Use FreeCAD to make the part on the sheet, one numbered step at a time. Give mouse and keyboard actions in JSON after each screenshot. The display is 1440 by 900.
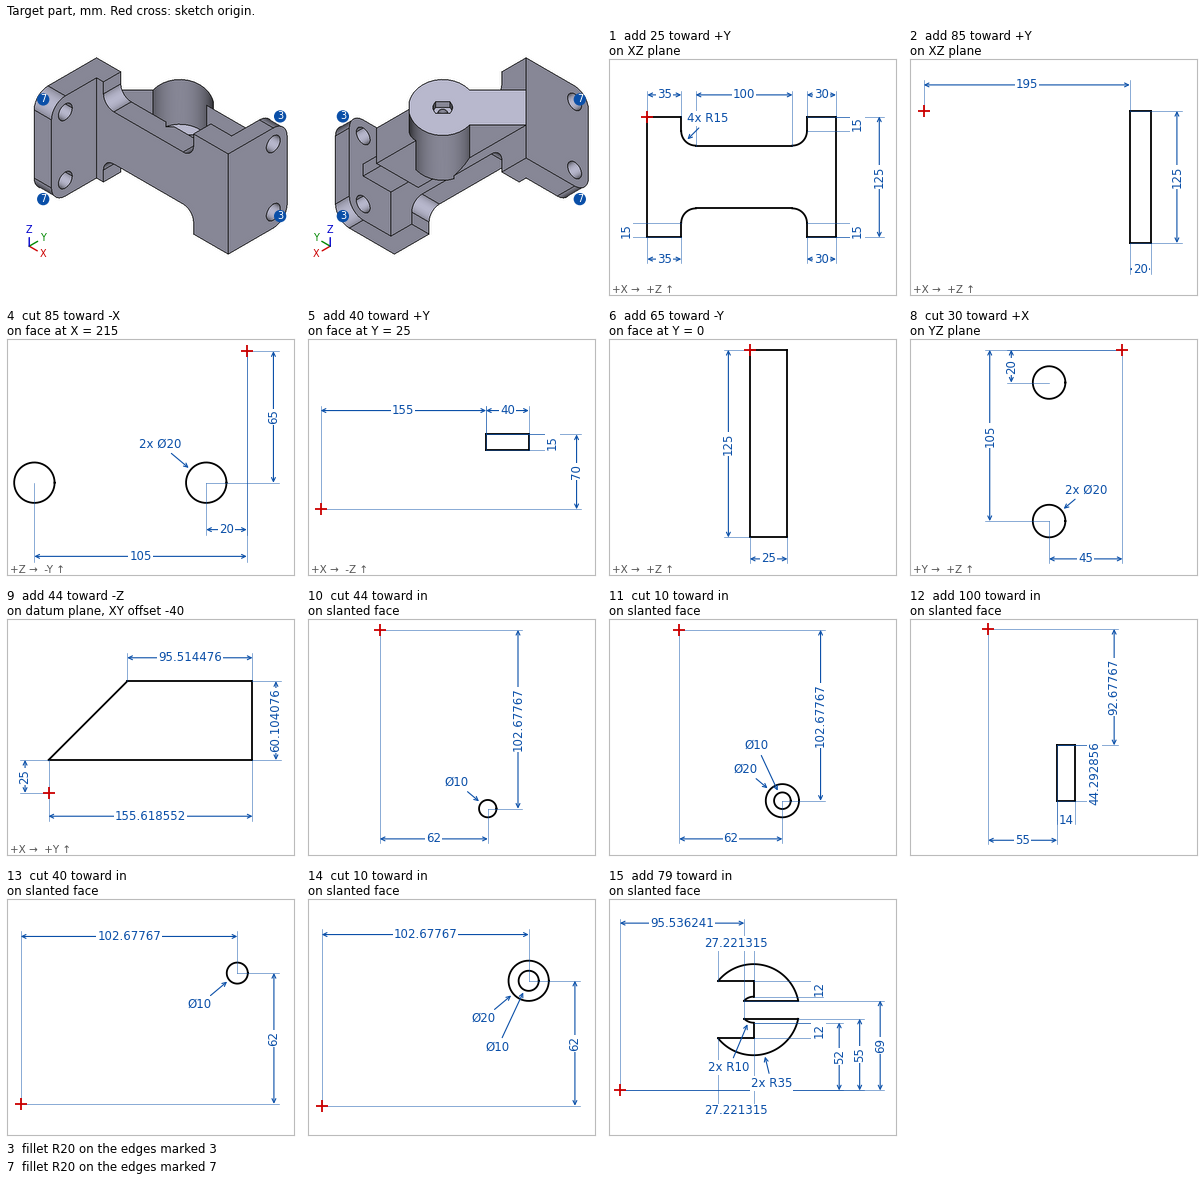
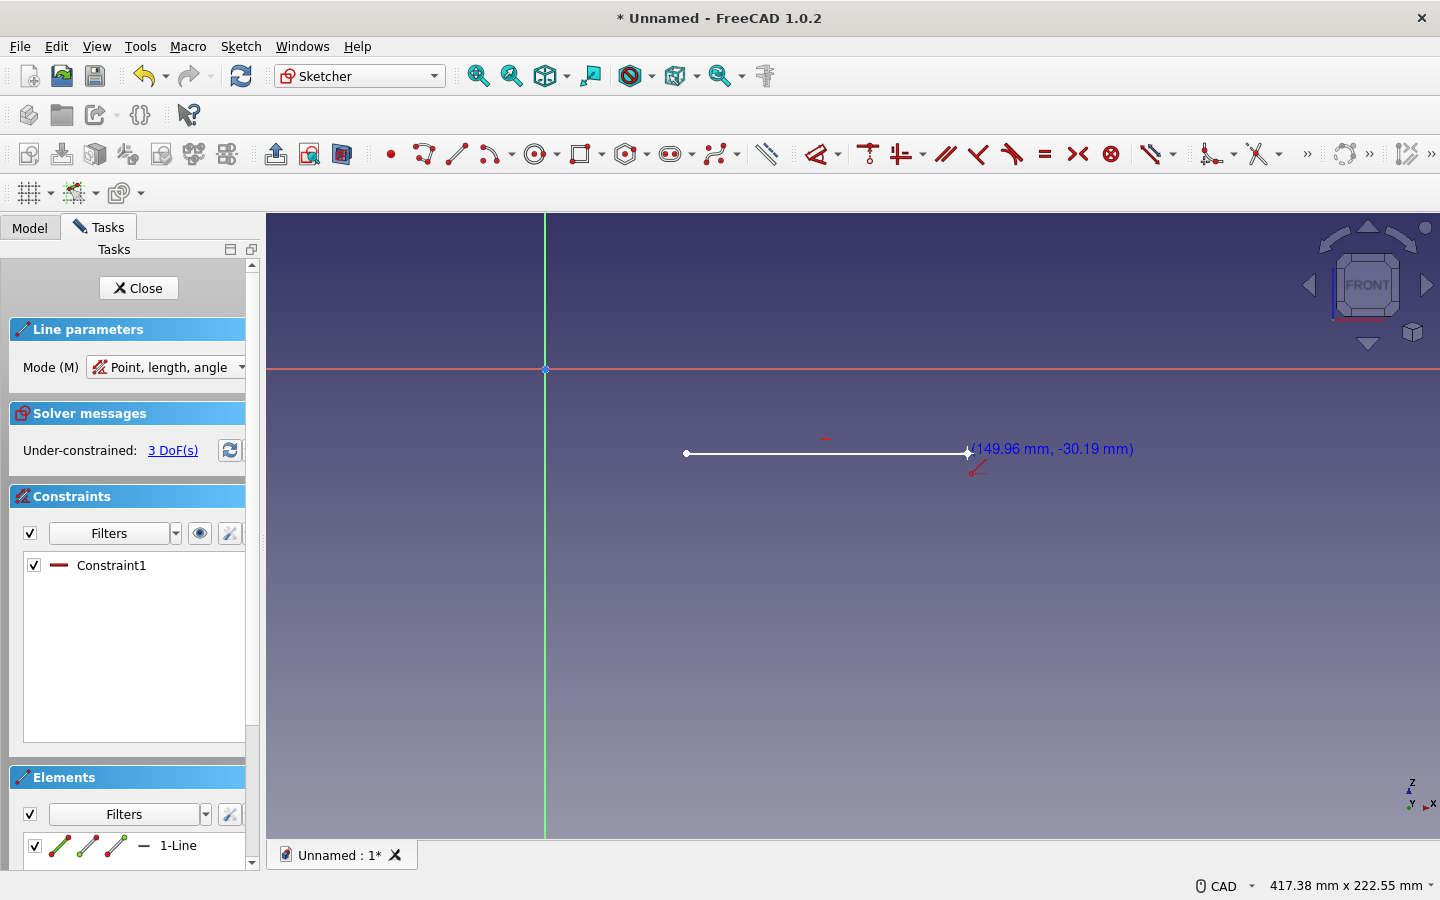
{"action": "left_click", "coordinate": [424, 154]}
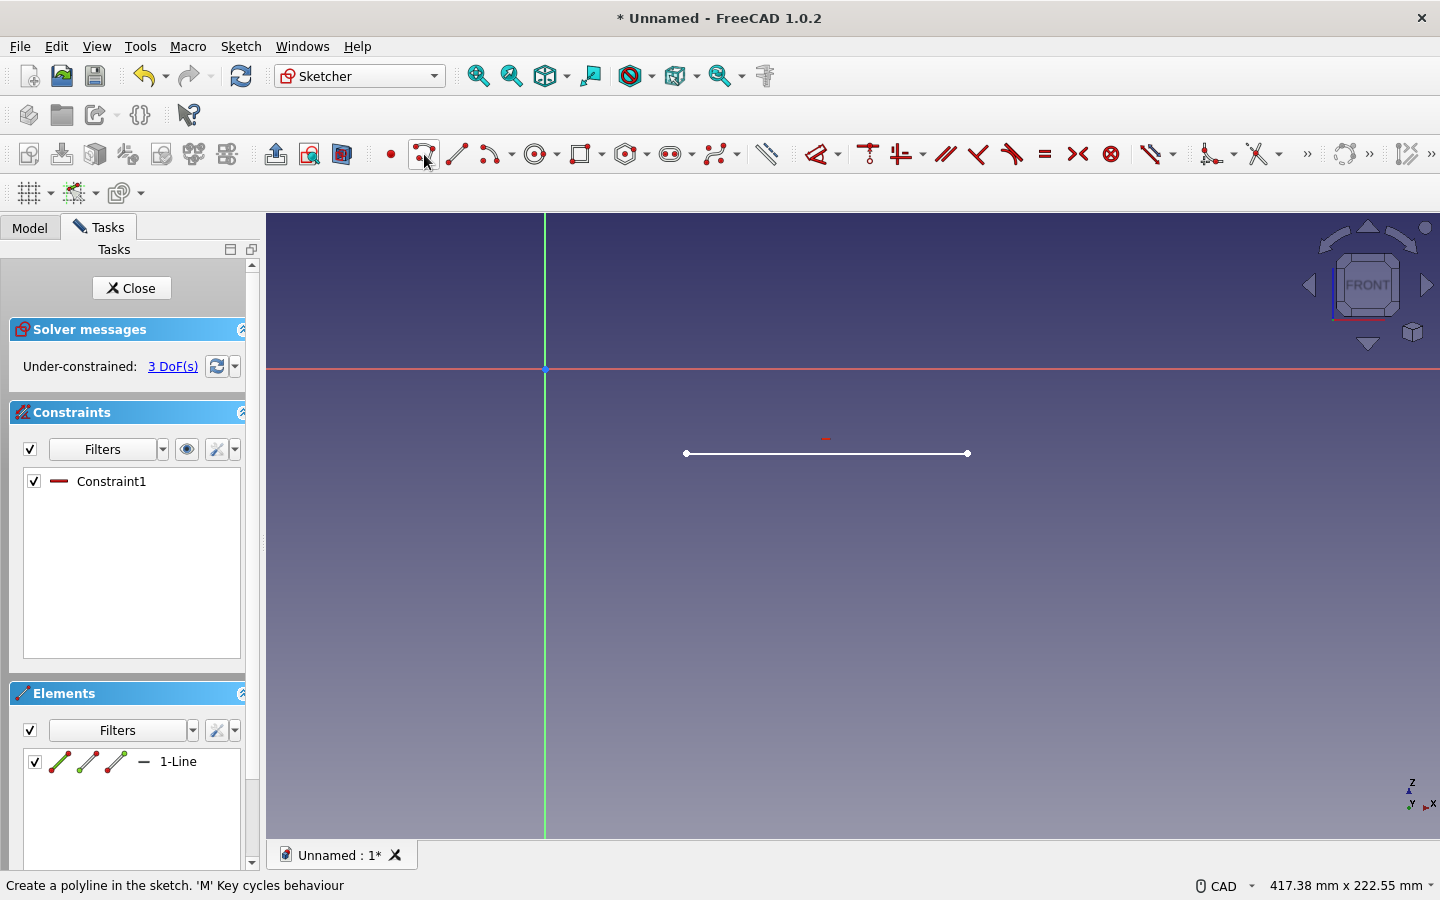
{"action": "left_click", "coordinate": [1009, 411]}
{"action": "left_click", "coordinate": [1009, 369]}
{"action": "left_click", "coordinate": [1094, 378]}
{"action": "left_click", "coordinate": [1094, 721]}
{"action": "left_click", "coordinate": [1009, 721]}
{"action": "left_click", "coordinate": [1009, 678]}
{"action": "right_click", "coordinate": [1009, 678]}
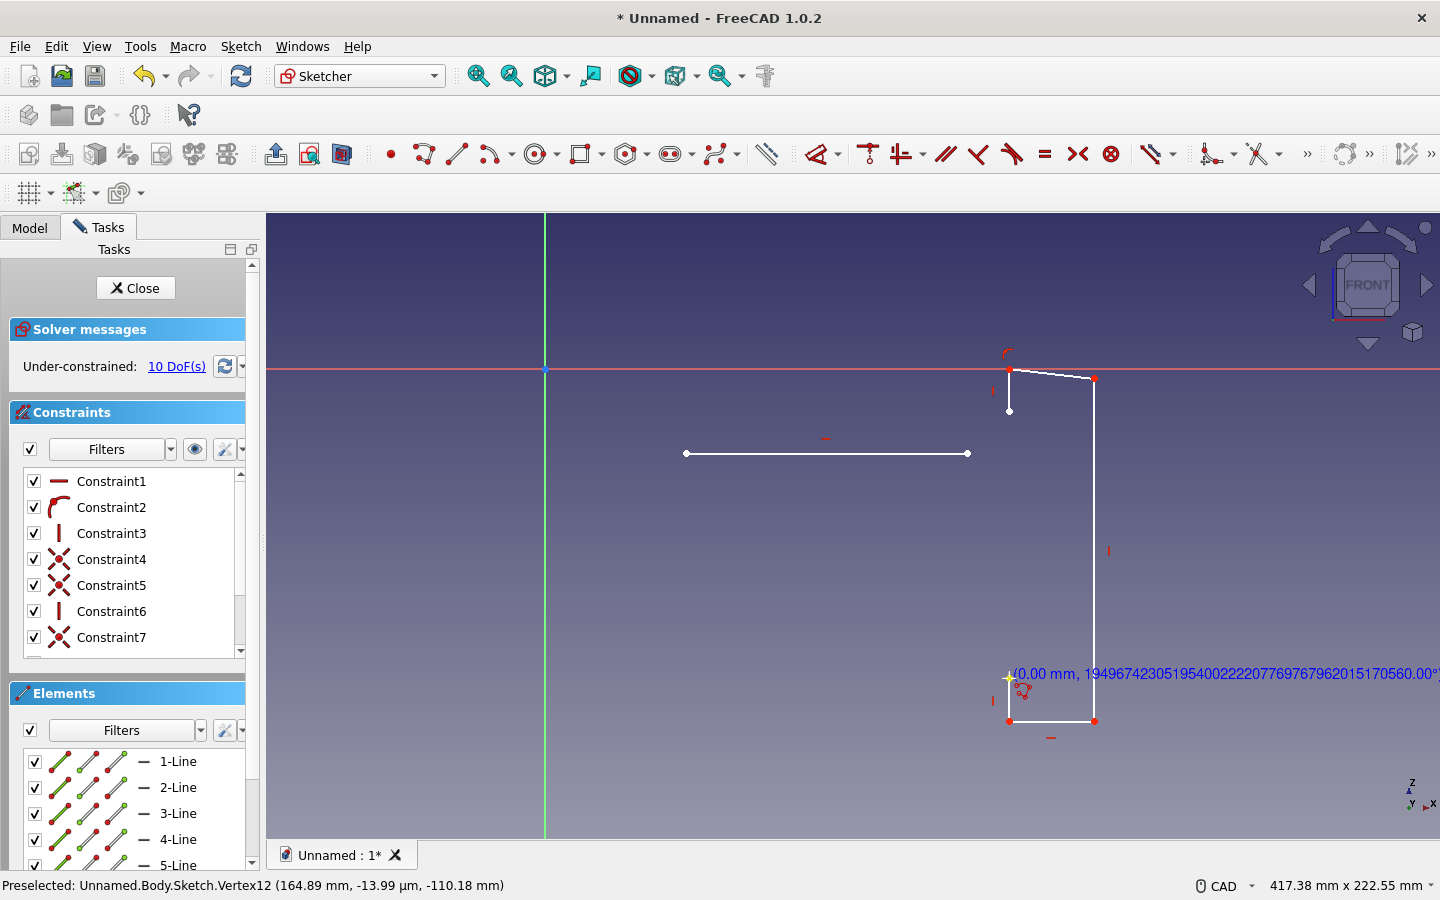
{"action": "left_click", "coordinate": [457, 154]}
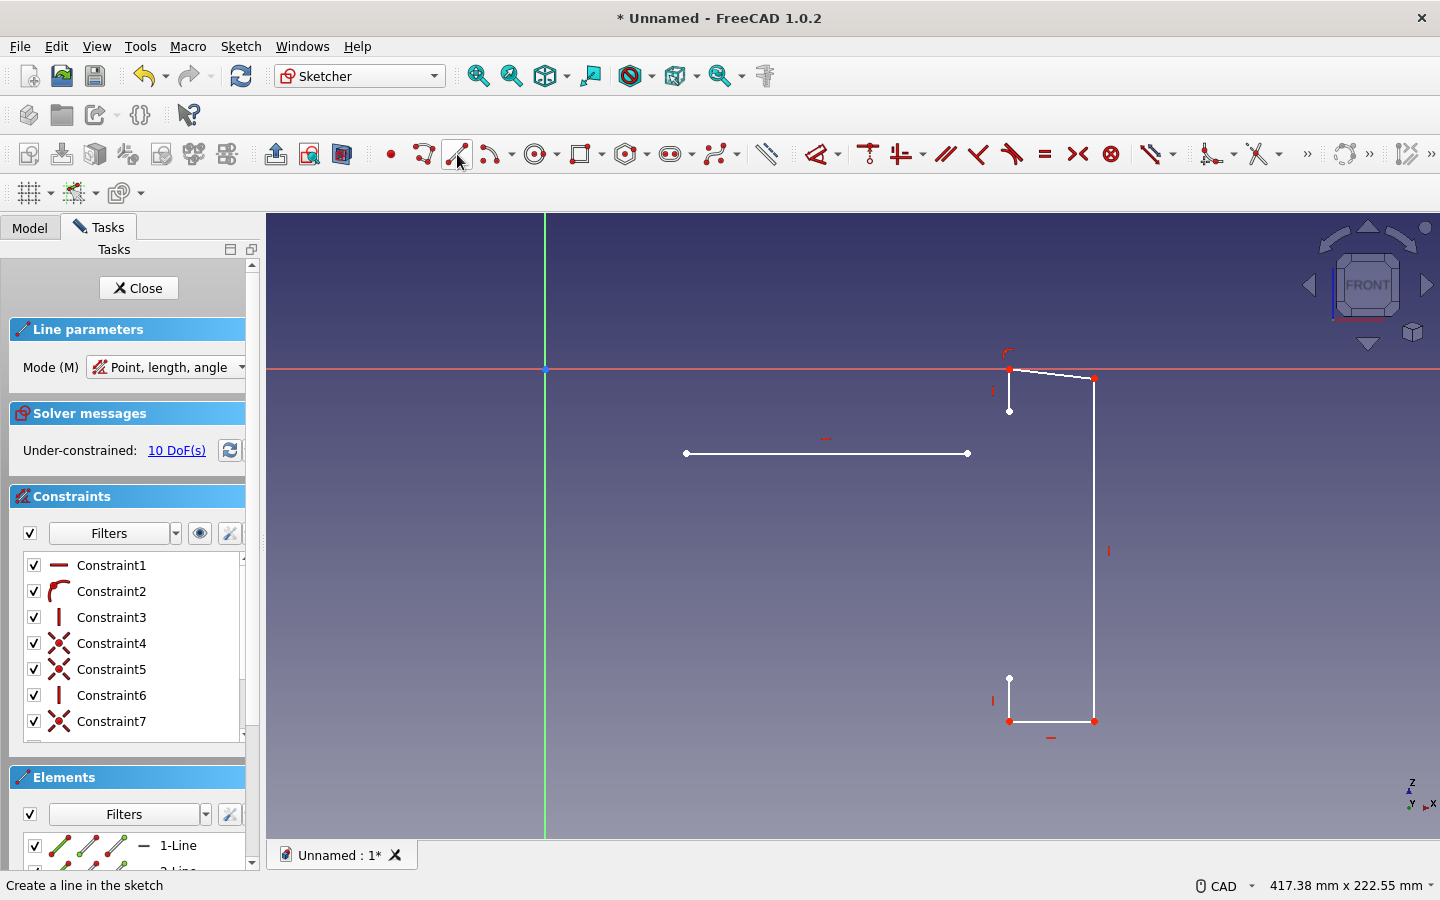
{"action": "left_click", "coordinate": [967, 636]}
{"action": "left_click", "coordinate": [686, 636]}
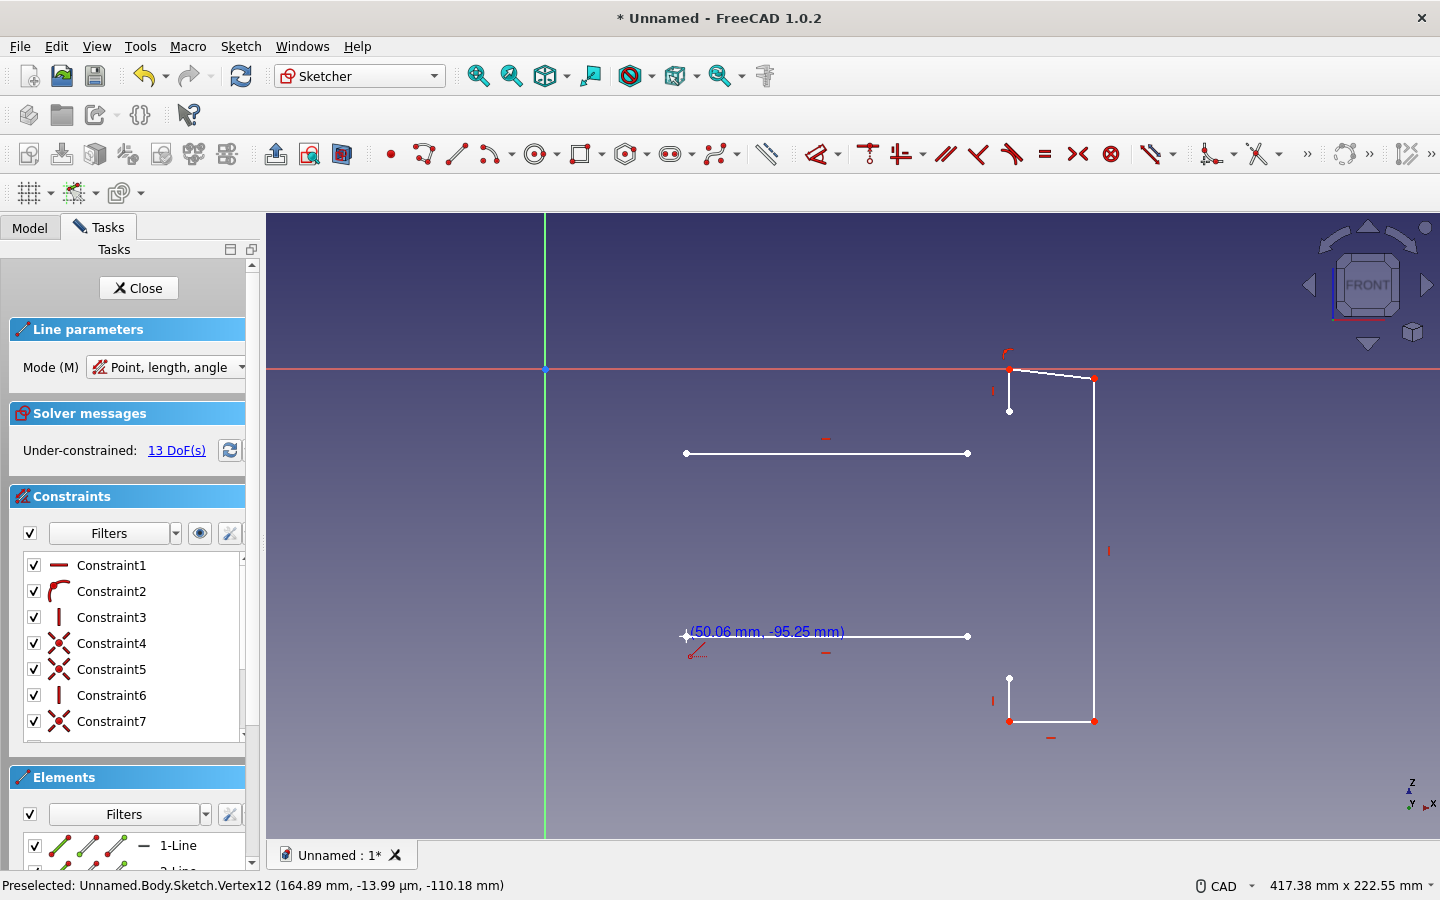
{"action": "left_click", "coordinate": [424, 154]}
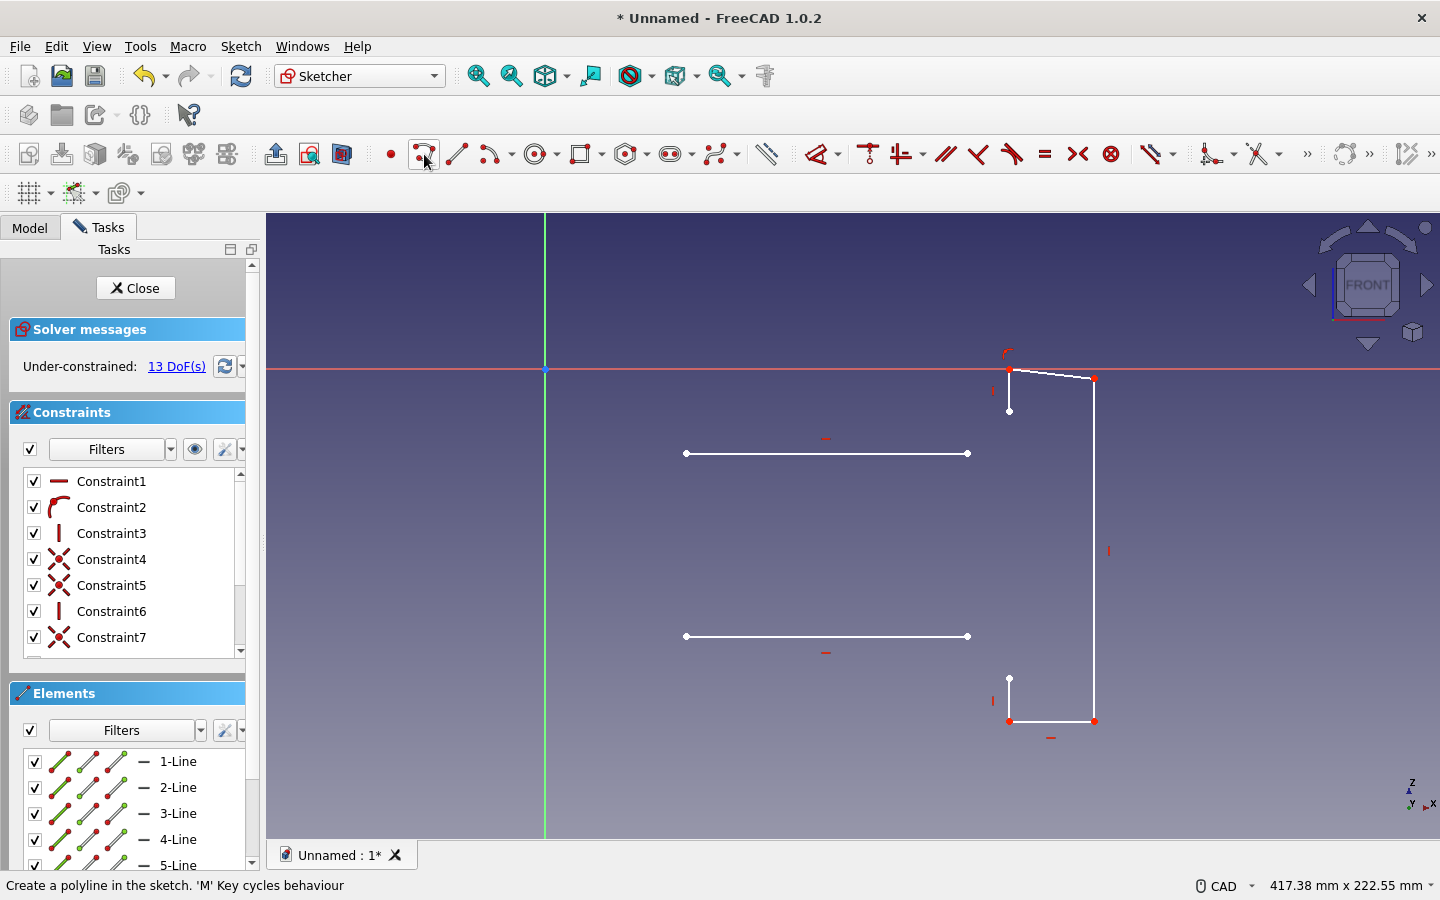
{"action": "left_click", "coordinate": [644, 678]}
{"action": "left_click", "coordinate": [644, 721]}
{"action": "left_click", "coordinate": [545, 721]}
{"action": "left_click", "coordinate": [545, 369]}
{"action": "left_click", "coordinate": [644, 378]}
{"action": "left_click", "coordinate": [644, 411]}
{"action": "right_click", "coordinate": [644, 411]}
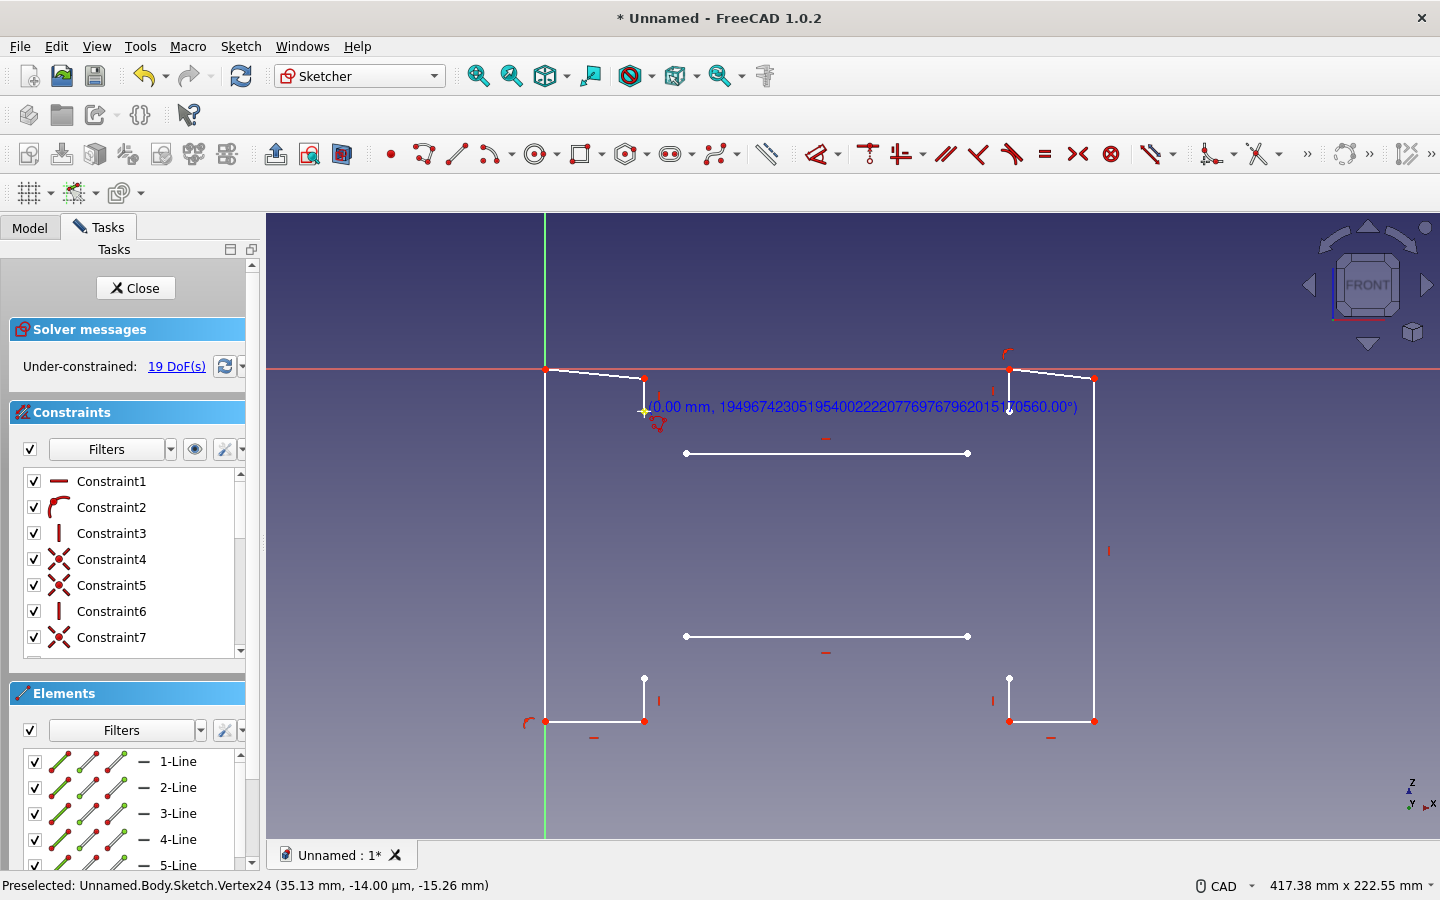
{"action": "left_click", "coordinate": [512, 154]}